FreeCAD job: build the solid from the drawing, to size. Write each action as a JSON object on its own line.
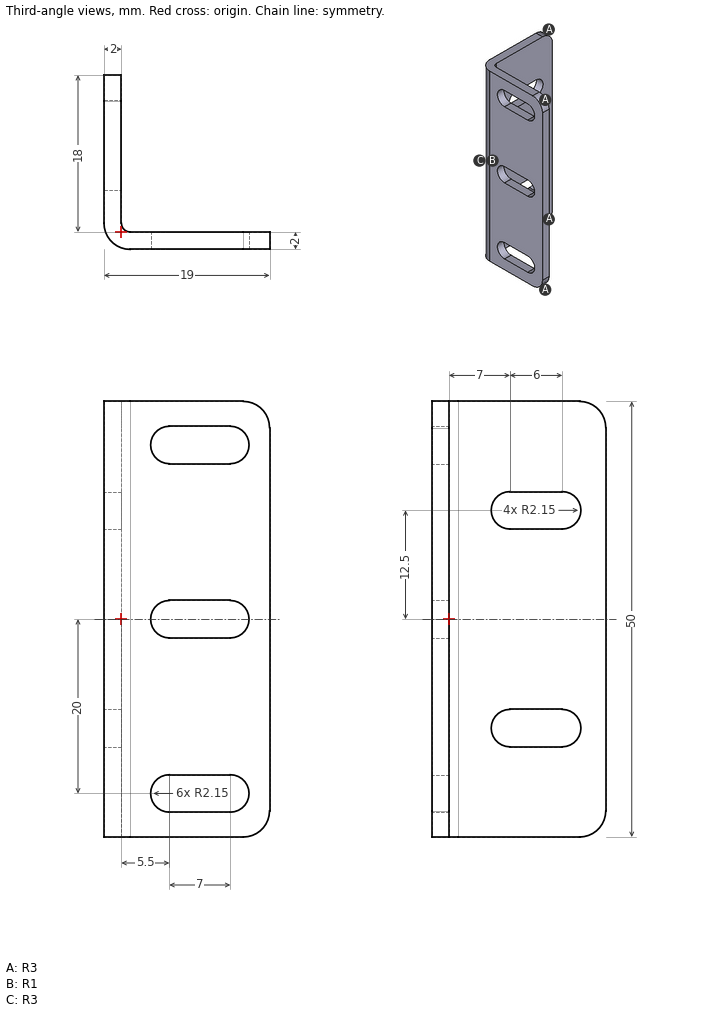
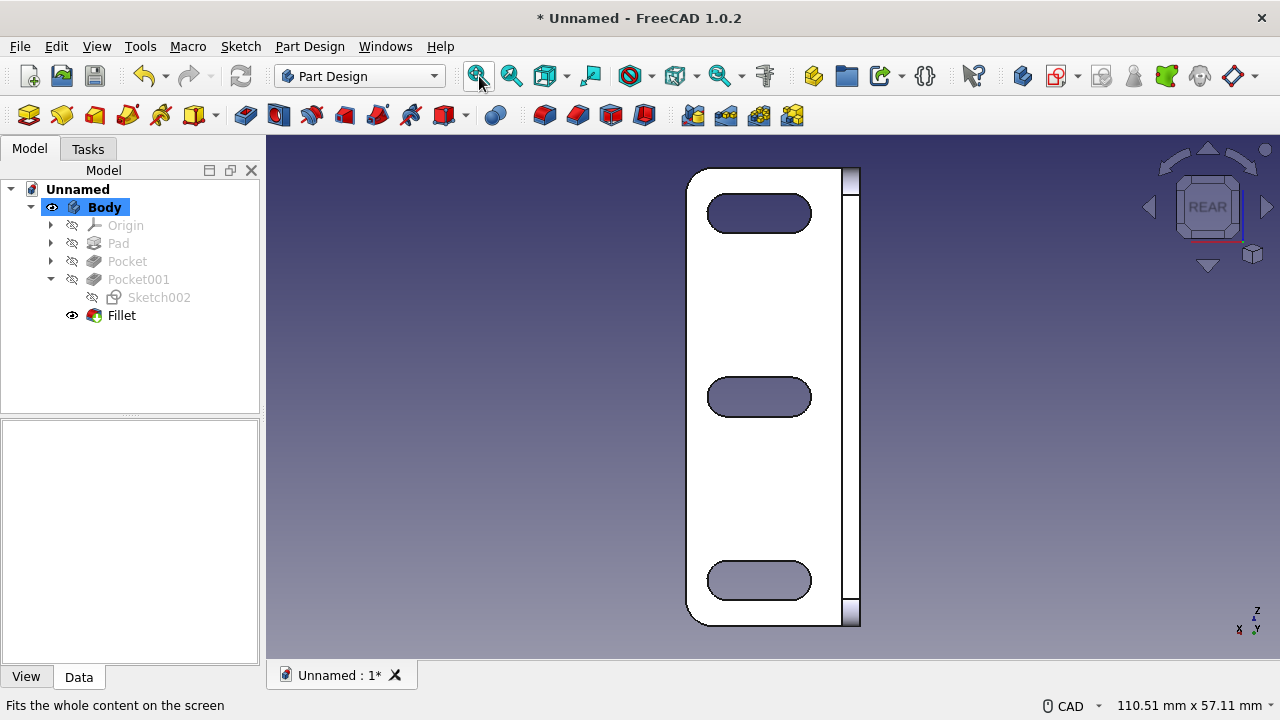
{"action": "key", "text": "6"}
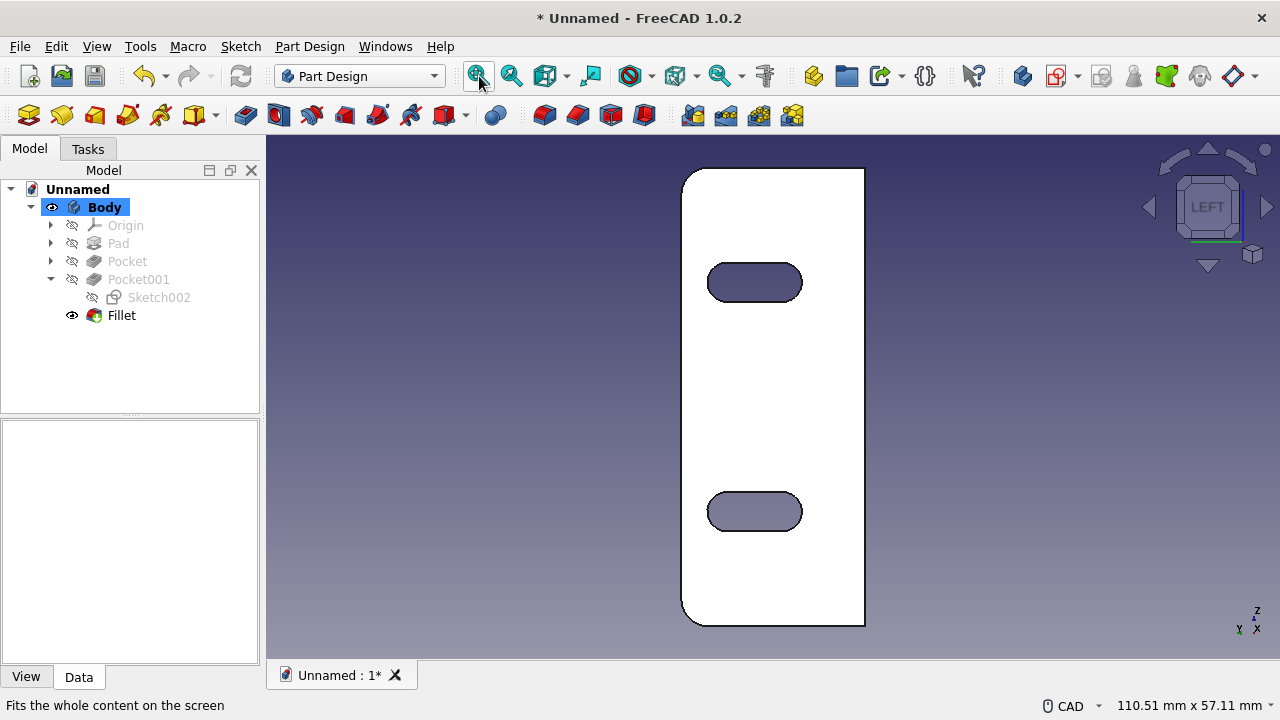
{"action": "key", "text": "v 3"}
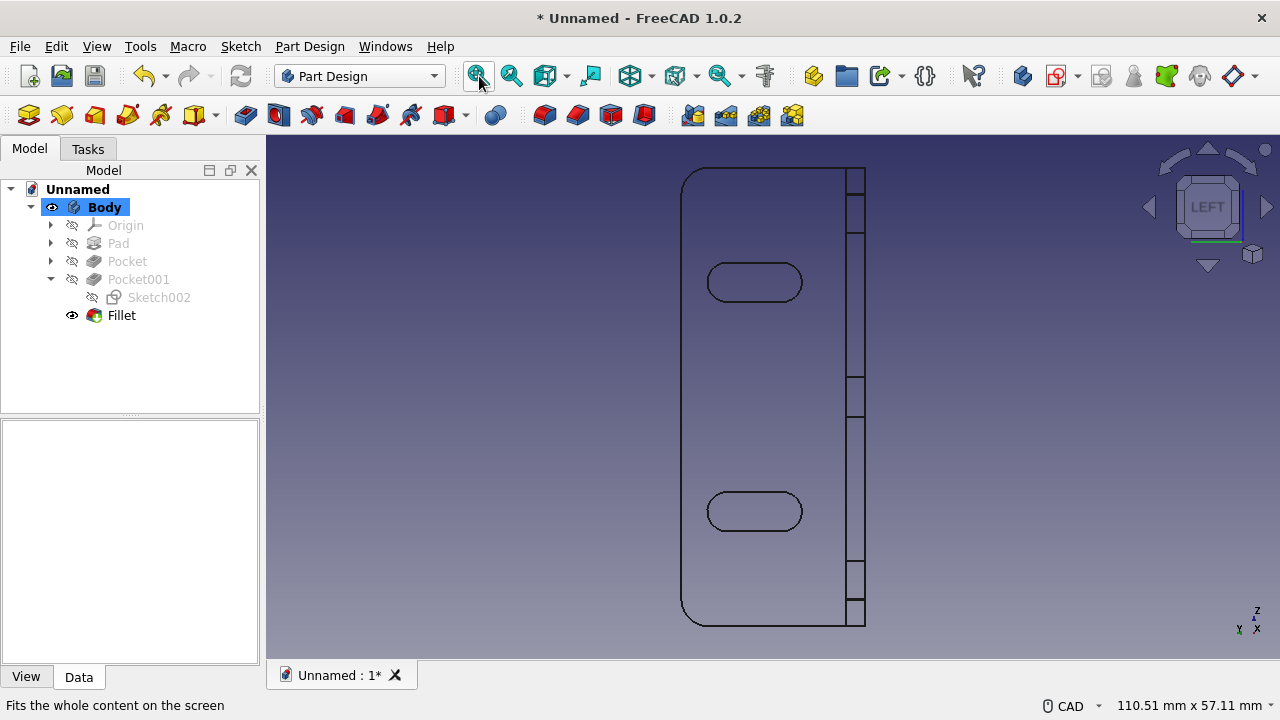
{"action": "key", "text": "0"}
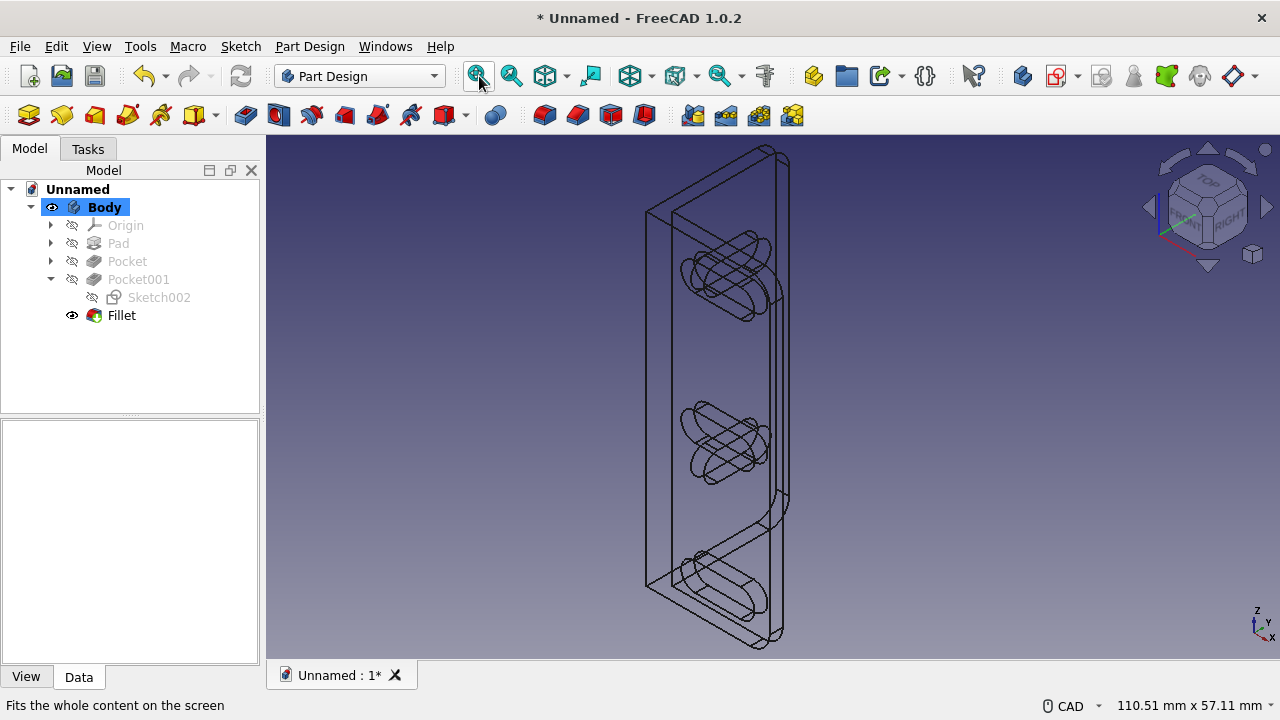
{"action": "left_click", "coordinate": [672, 398]}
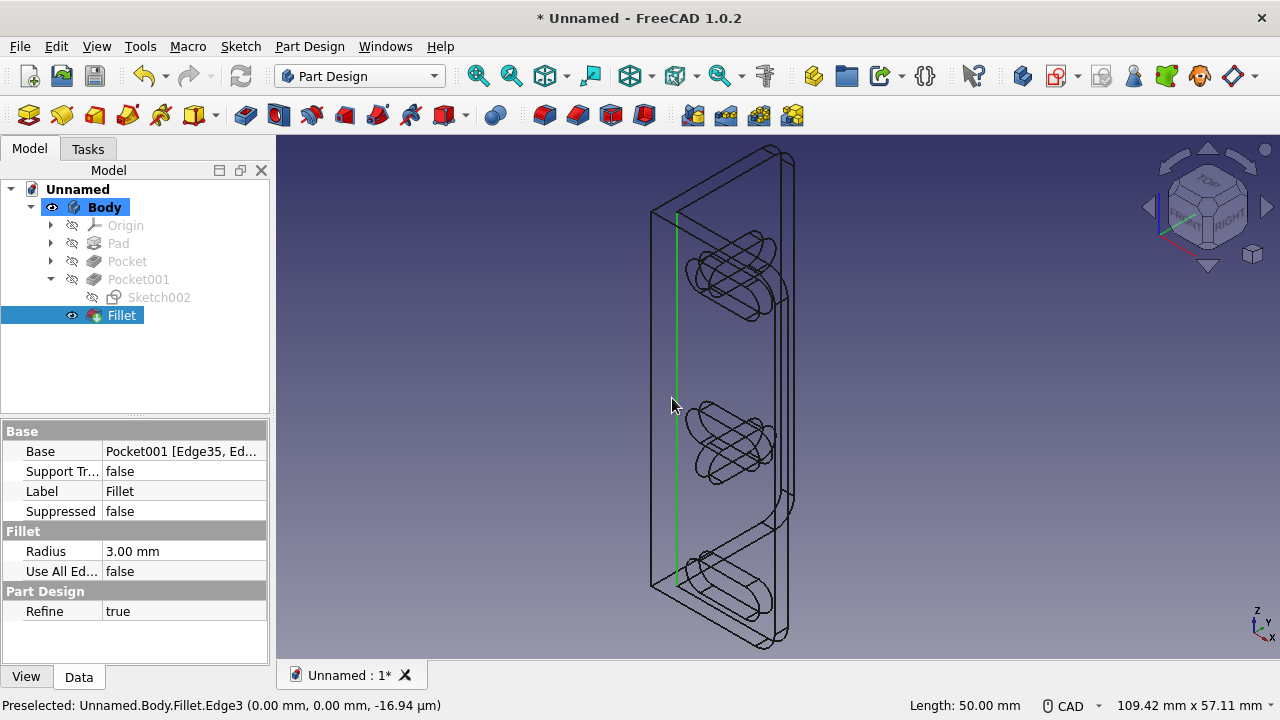
{"action": "key", "text": "v 1"}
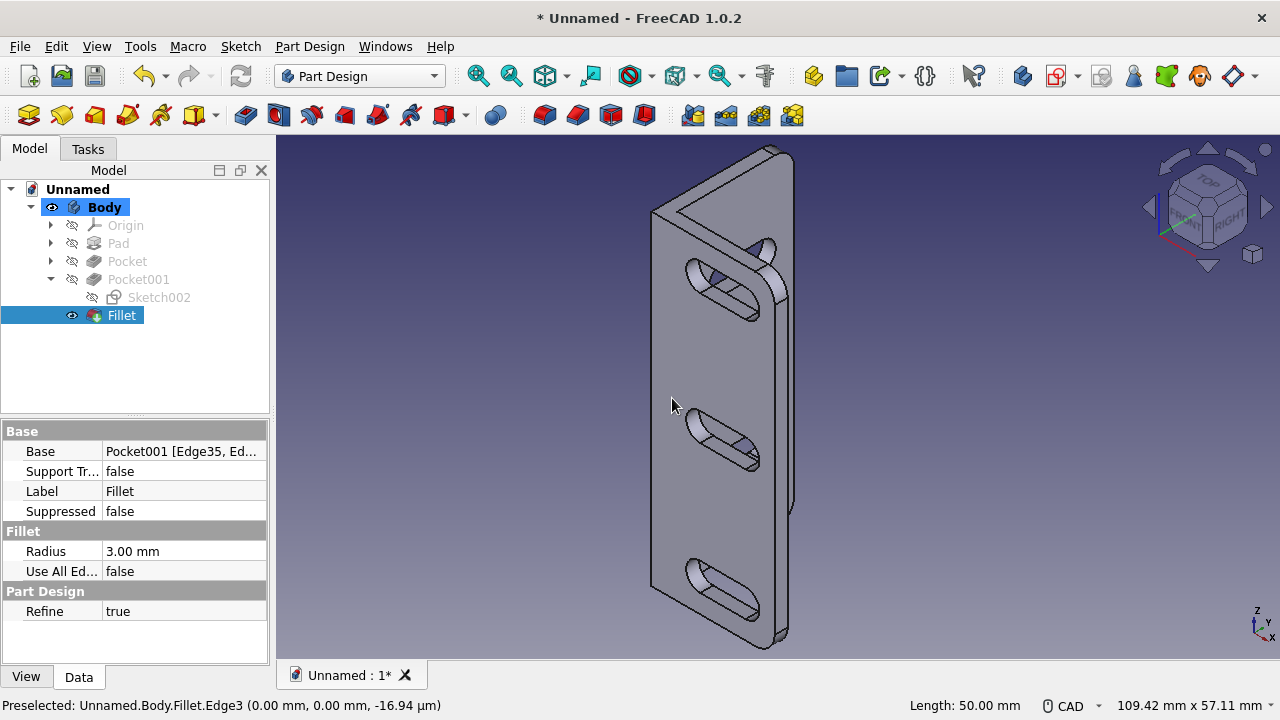
{"action": "left_click", "coordinate": [545, 116]}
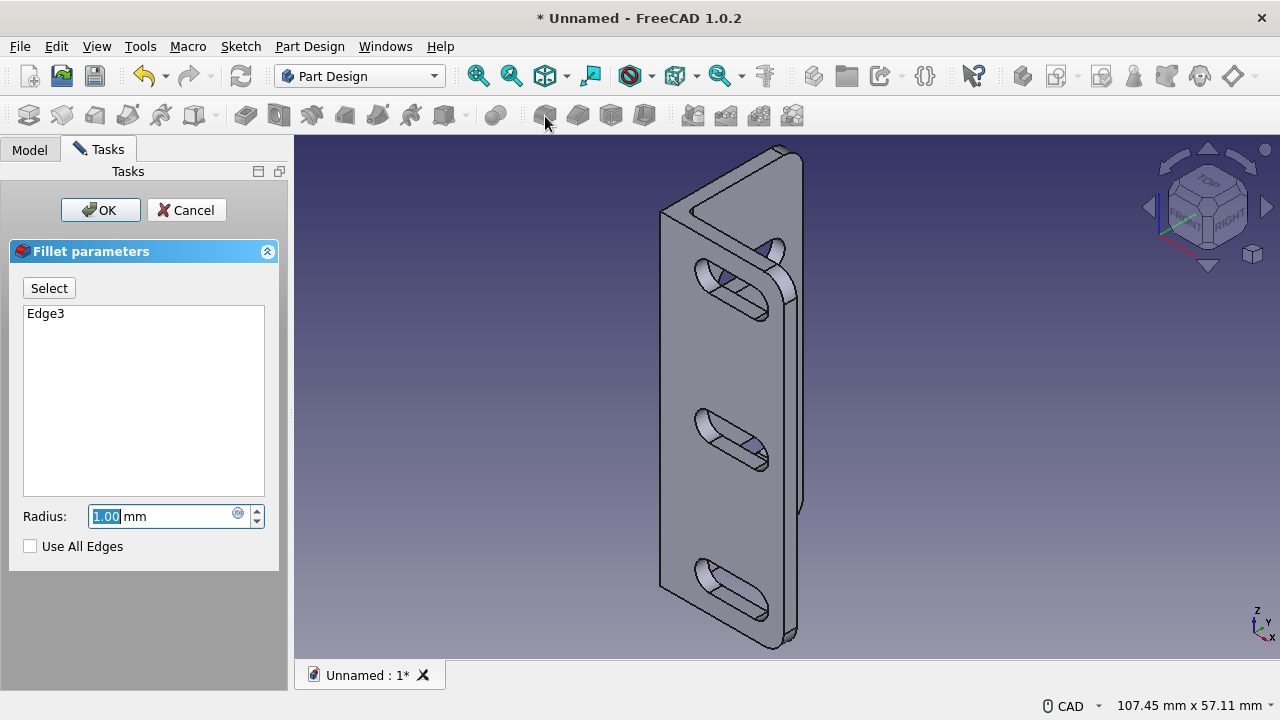
{"action": "type", "text": "1"}
{"action": "key", "text": "Tab"}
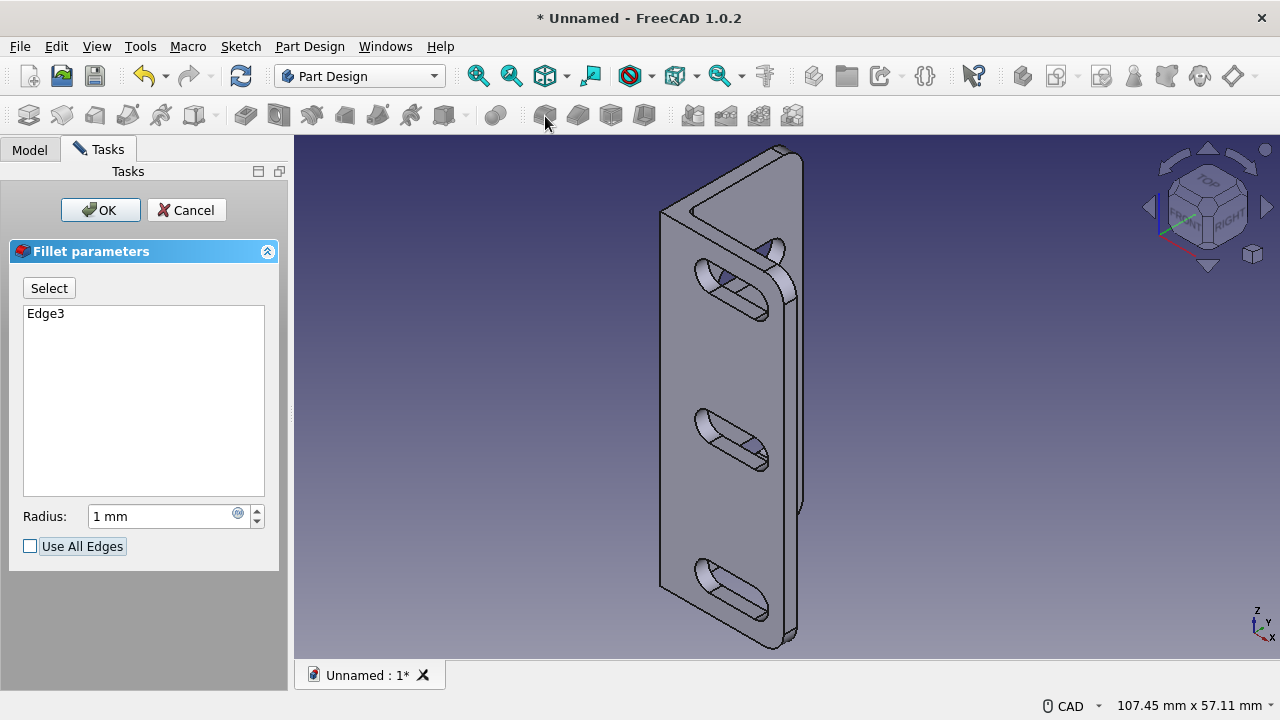
{"action": "left_click", "coordinate": [101, 210]}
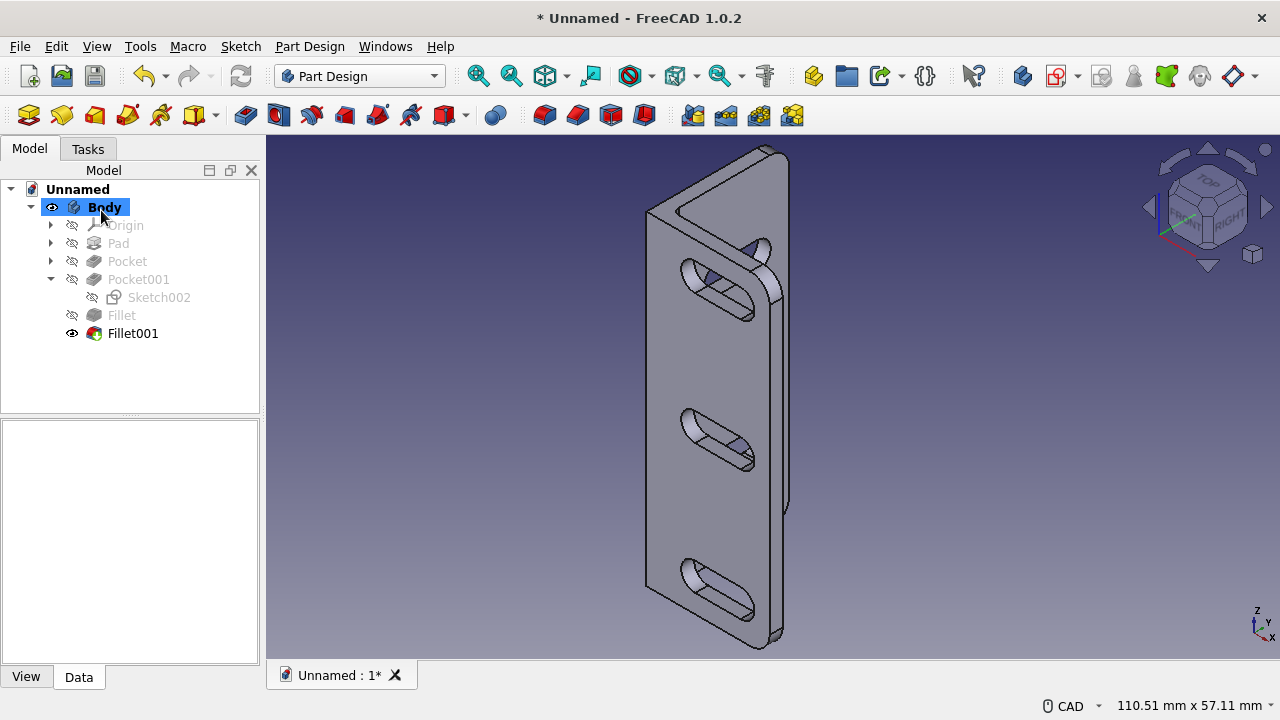
{"action": "key", "text": "2"}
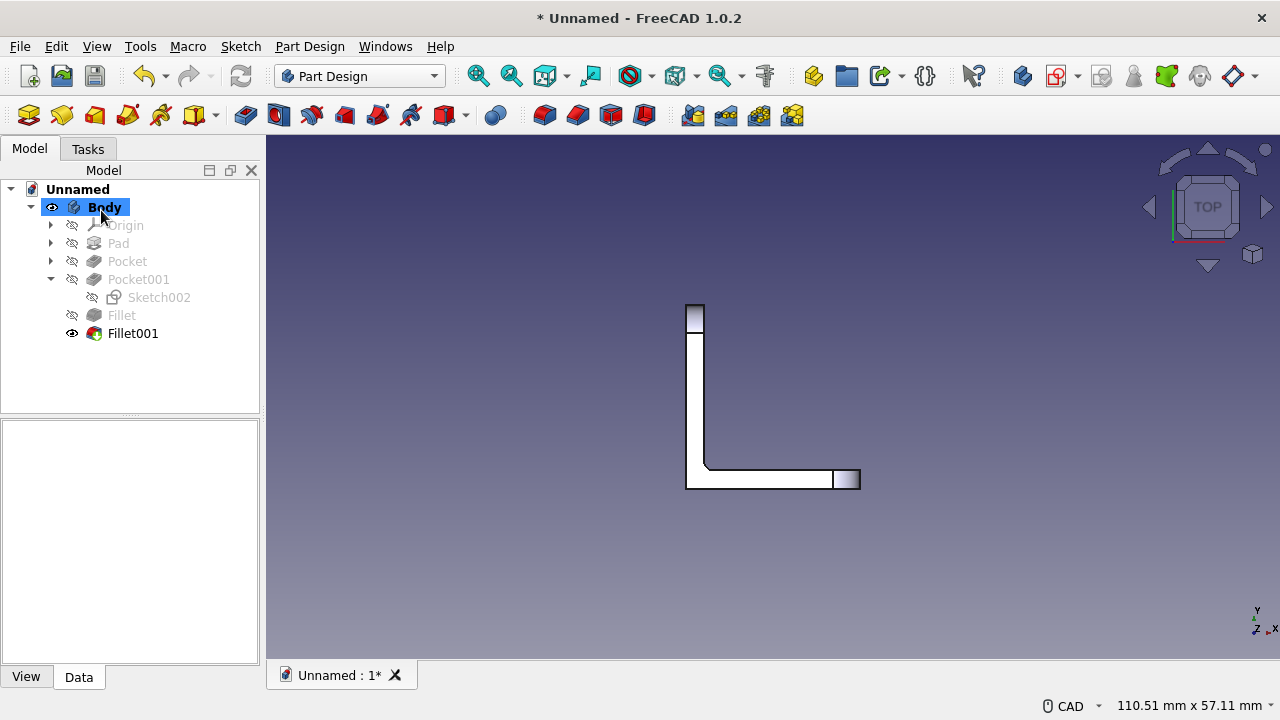
{"action": "left_click", "coordinate": [479, 76]}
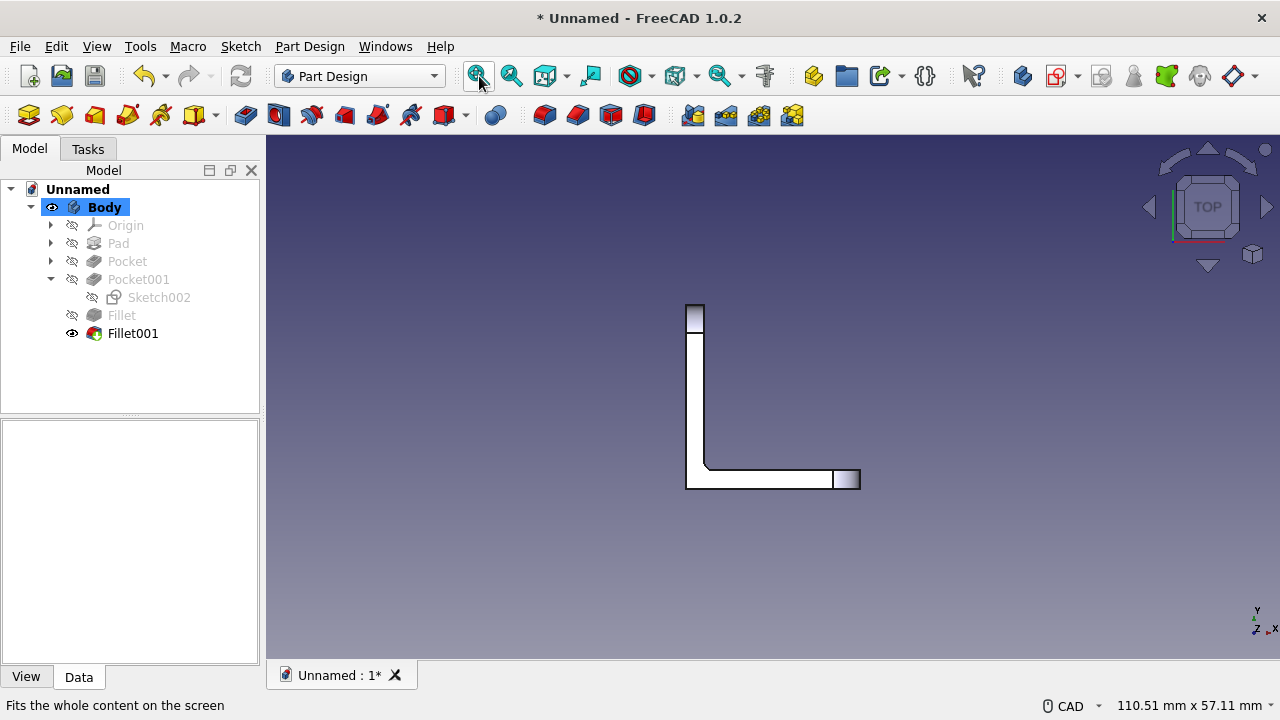
{"action": "key", "text": "0"}